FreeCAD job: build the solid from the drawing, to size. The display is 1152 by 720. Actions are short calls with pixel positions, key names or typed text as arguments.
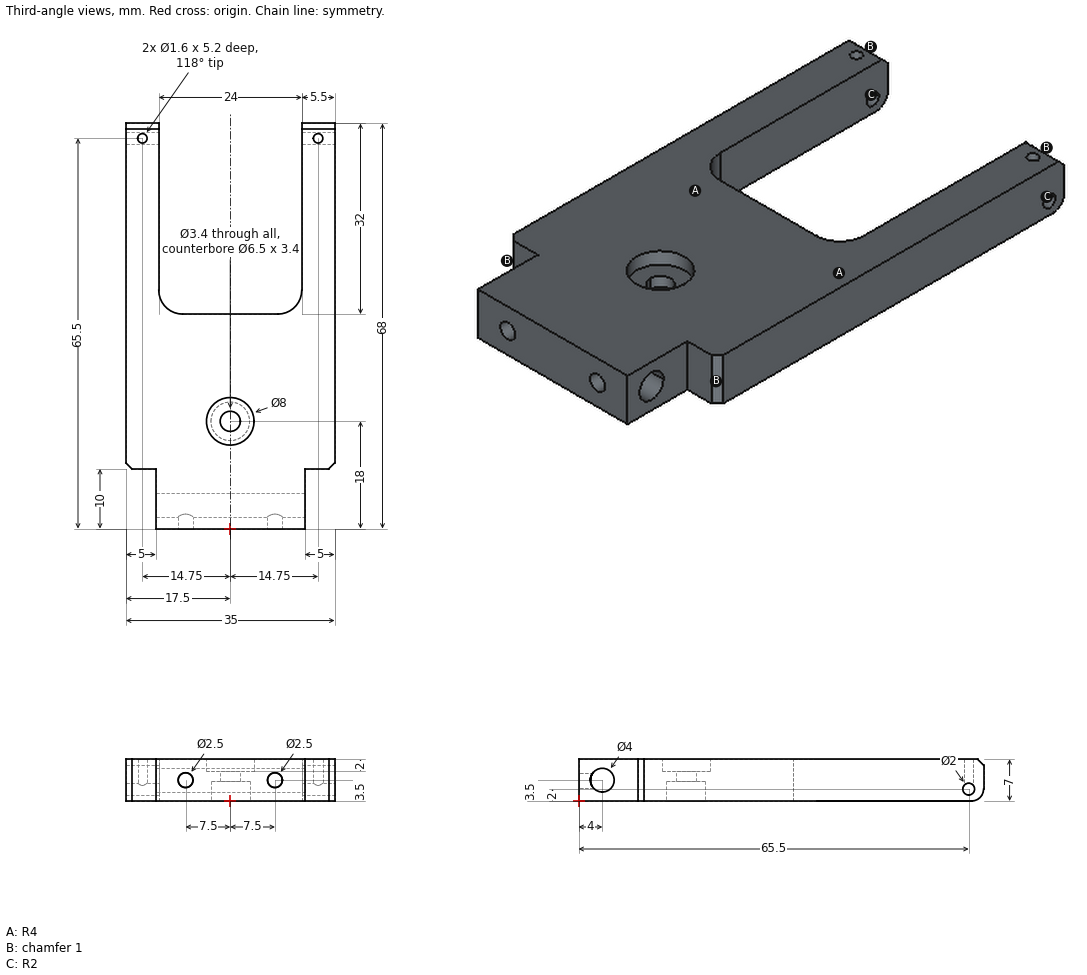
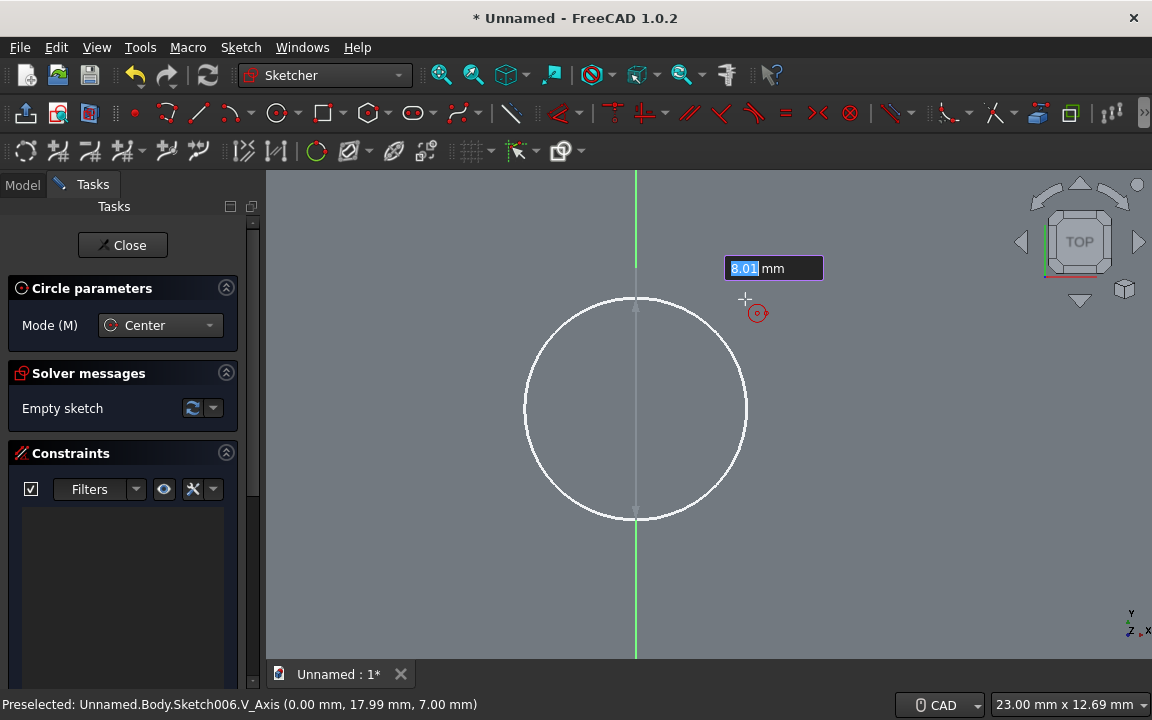
text(8)
key(Return)
key(Escape)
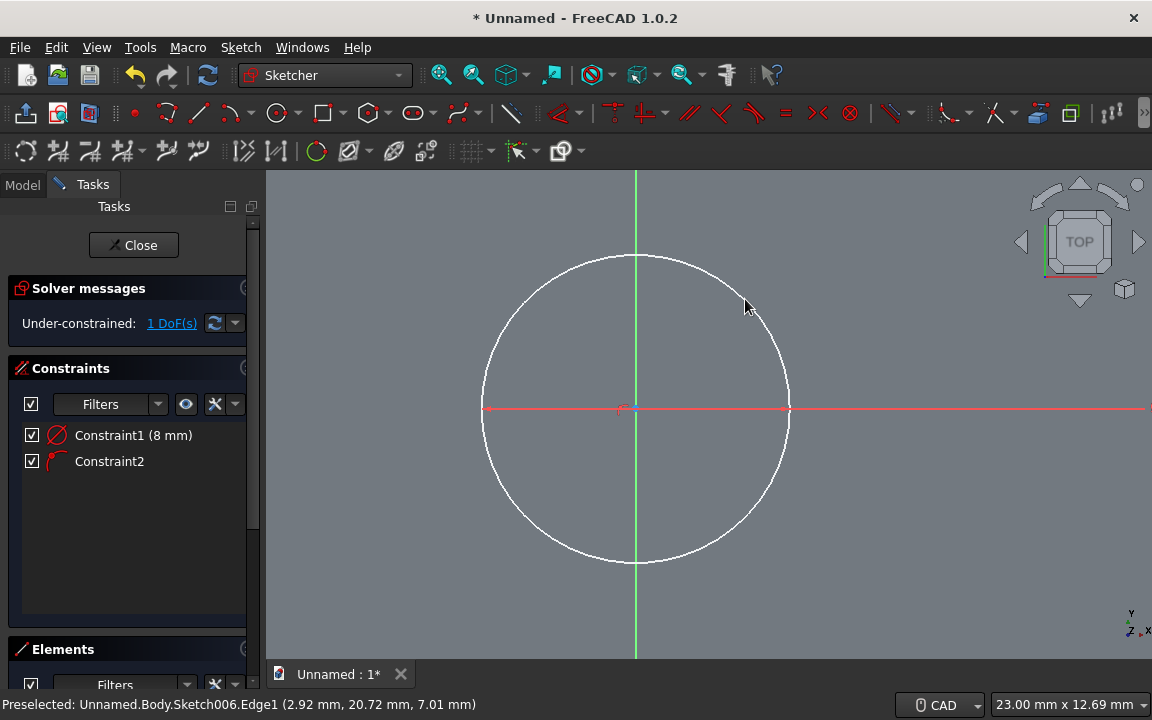
key(d)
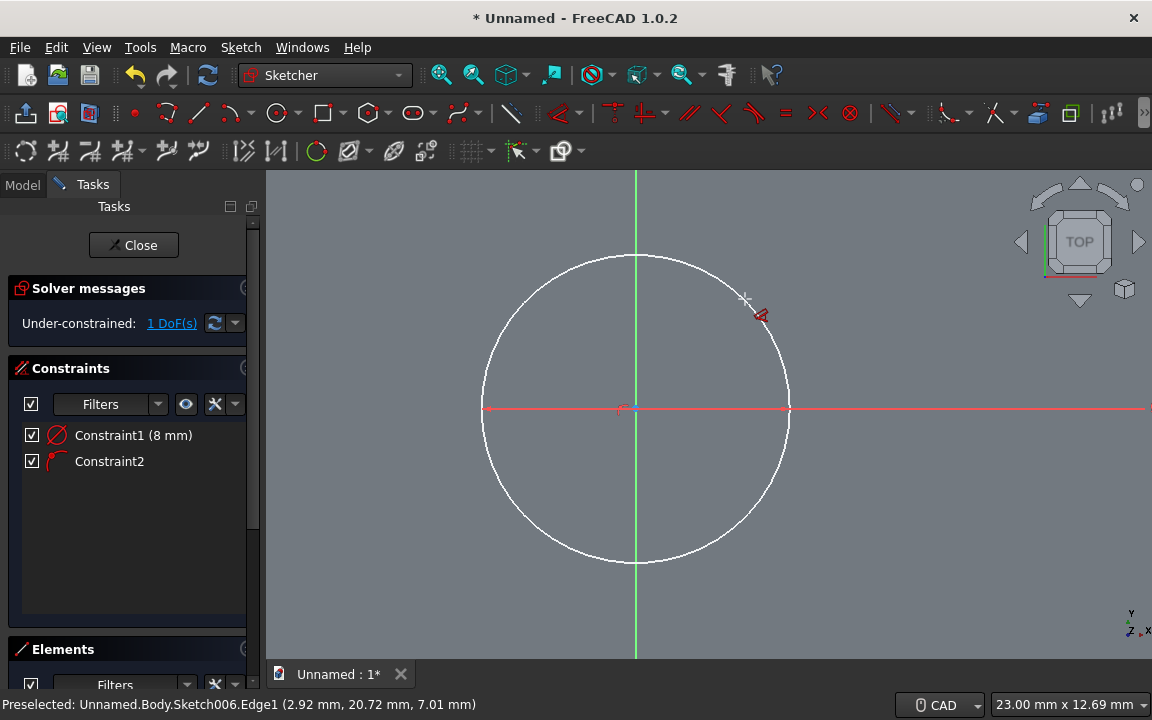
click(636, 409)
click(670, 520)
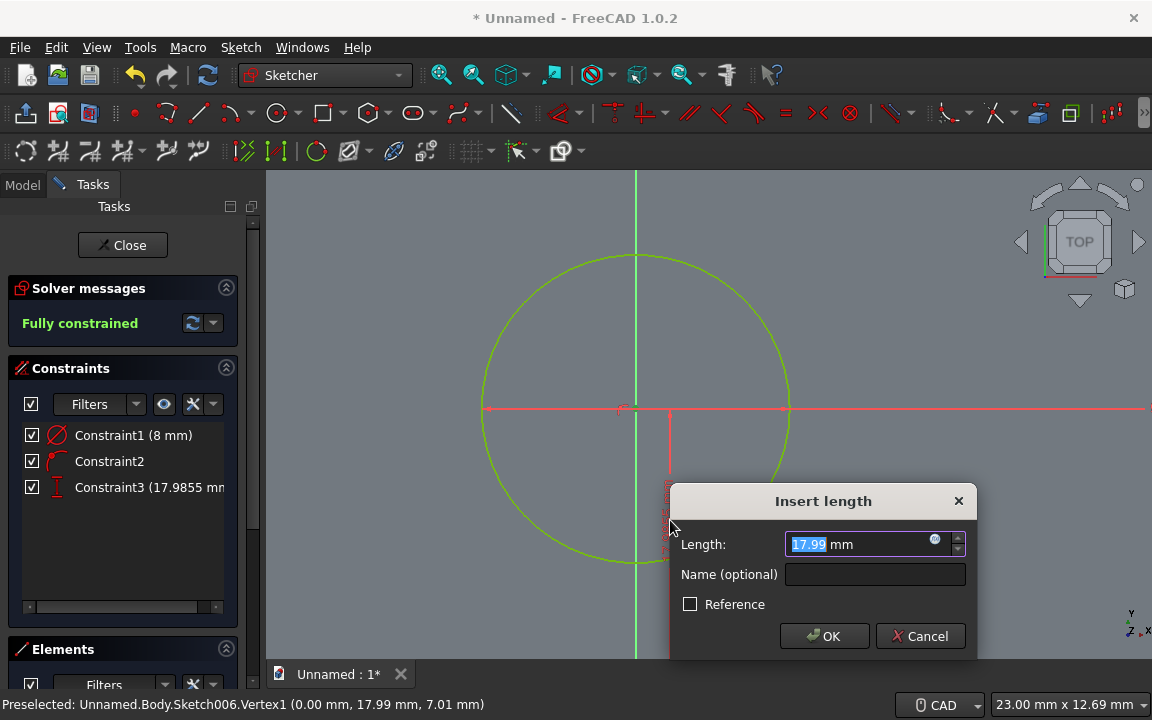
text(18)
key(Return)
key(Escape)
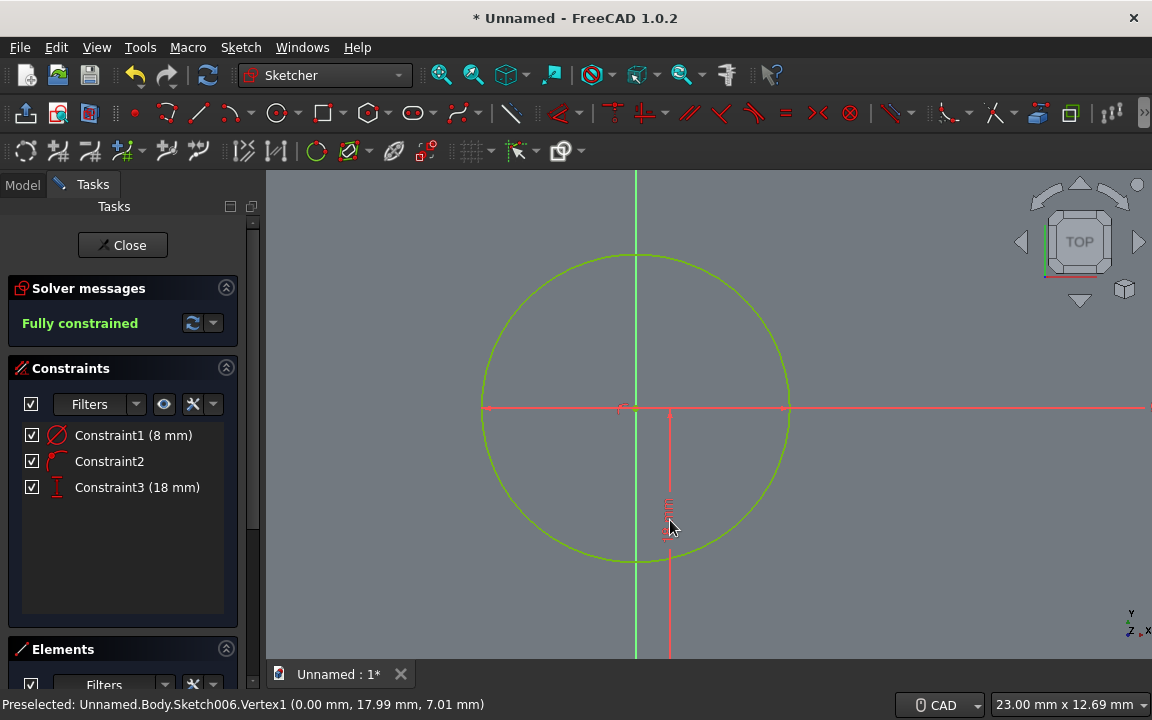
click(123, 245)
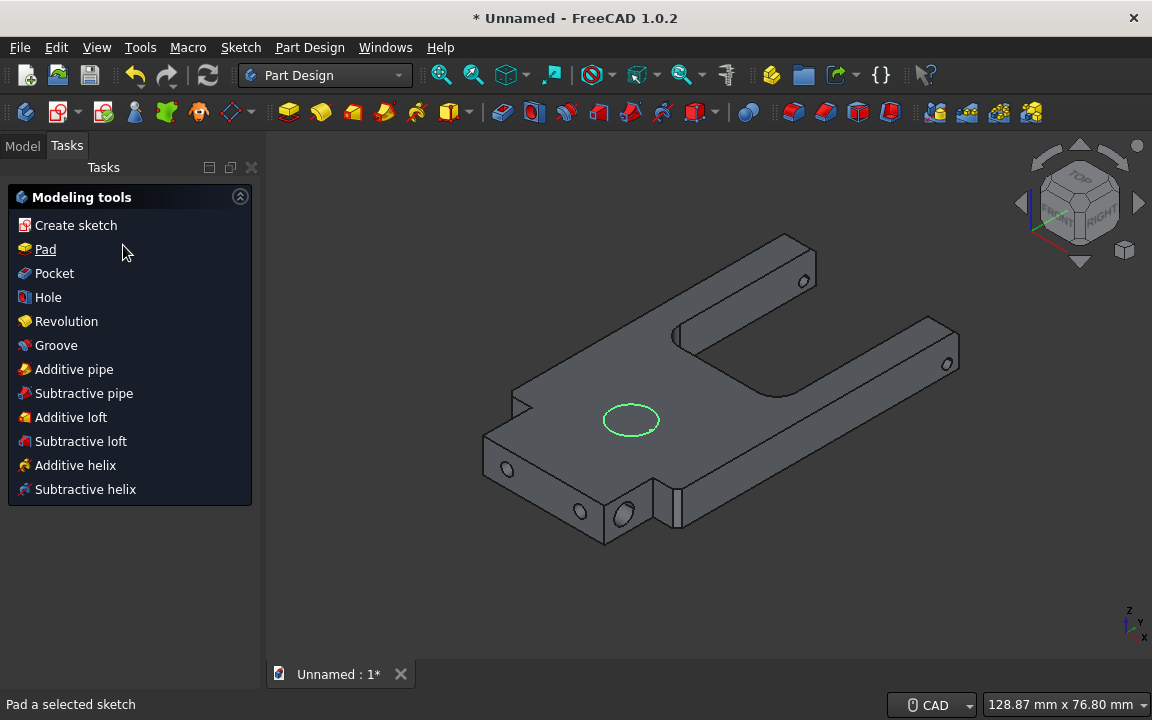
click(504, 112)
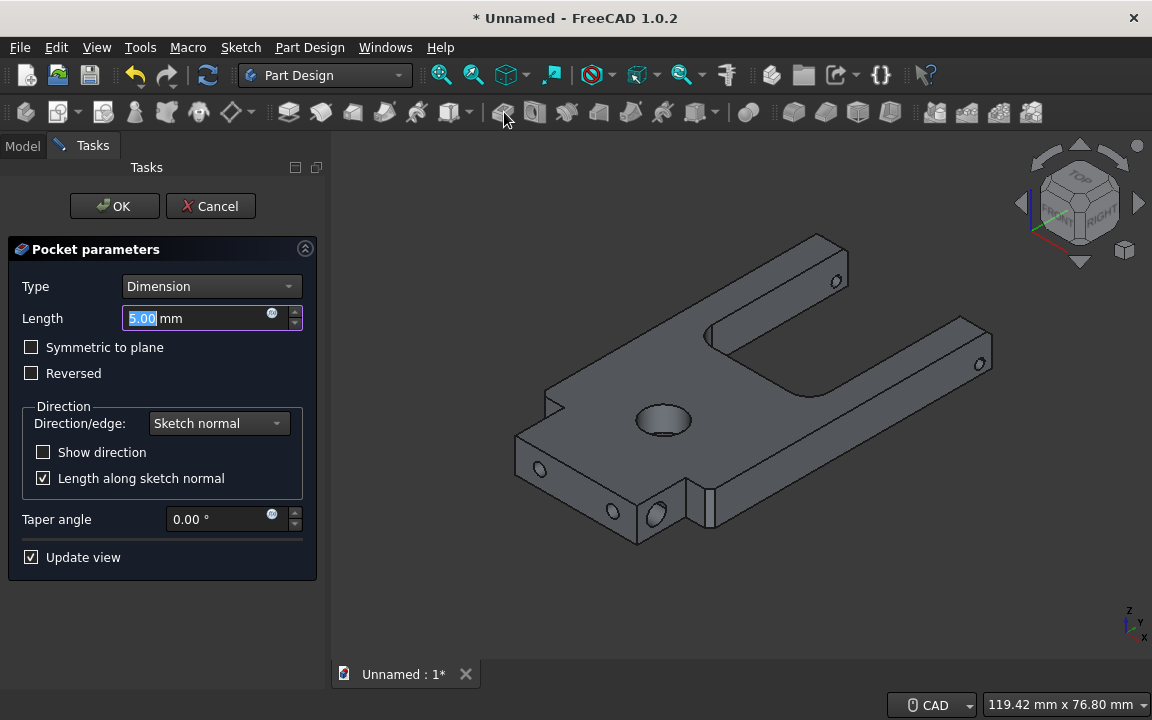
text(2)
key(Tab)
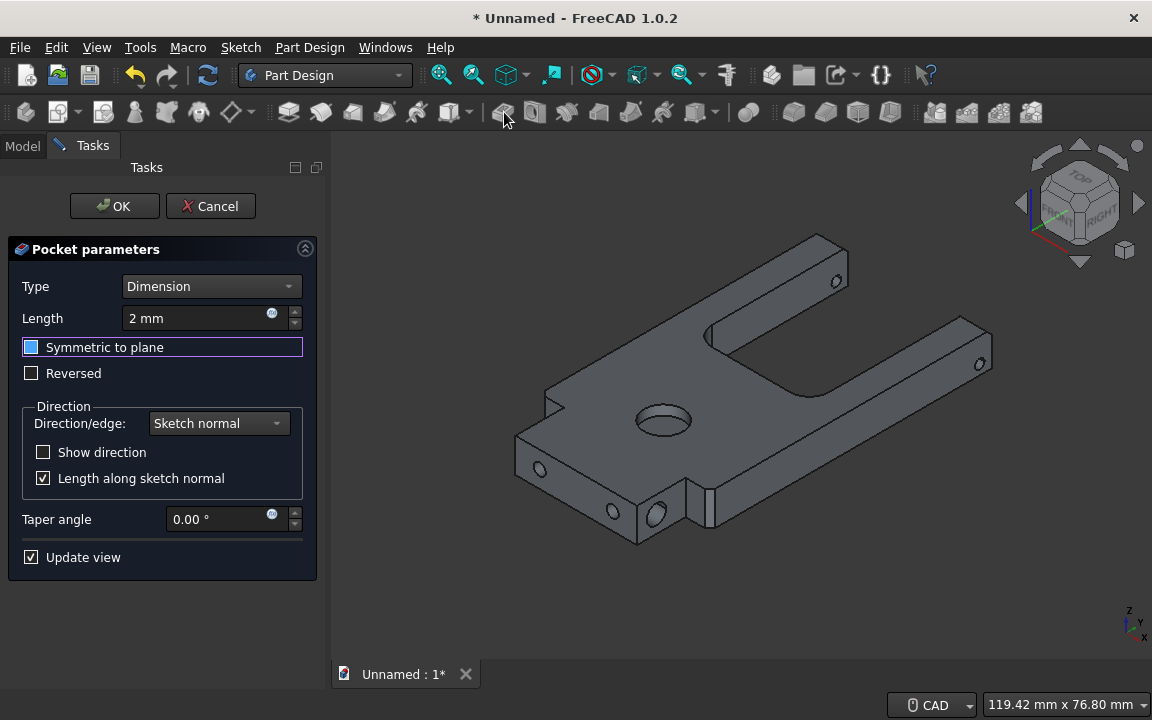
click(115, 206)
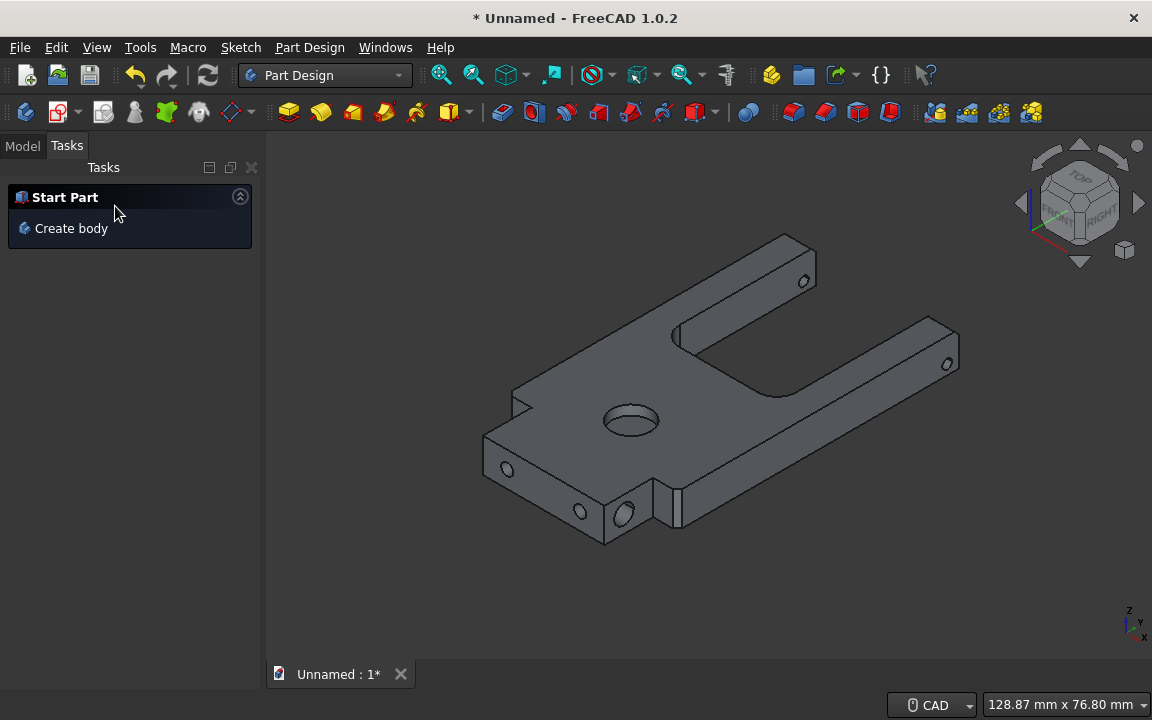
key(2)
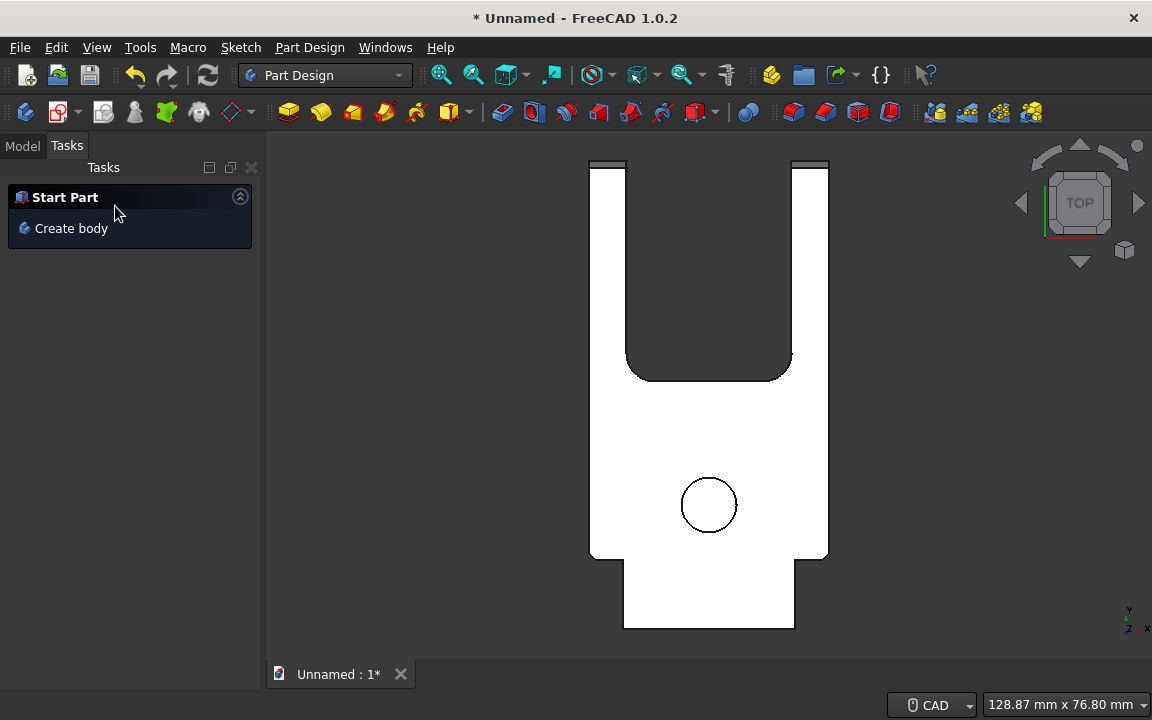
key(0)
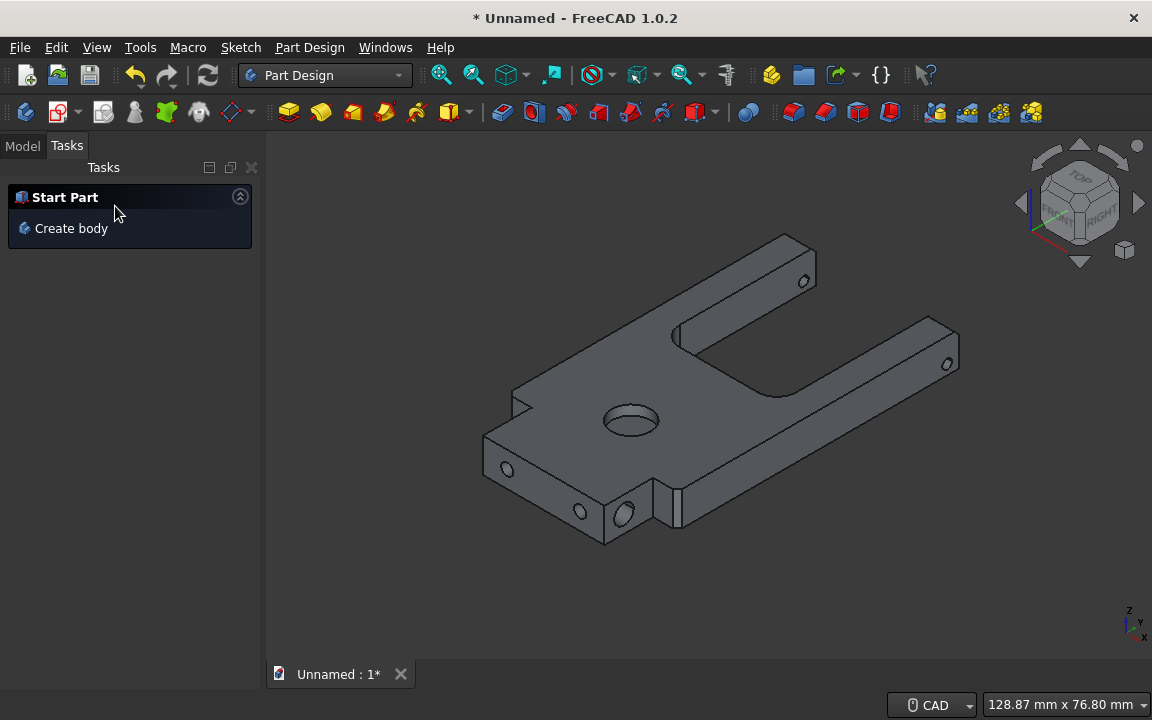
key(1)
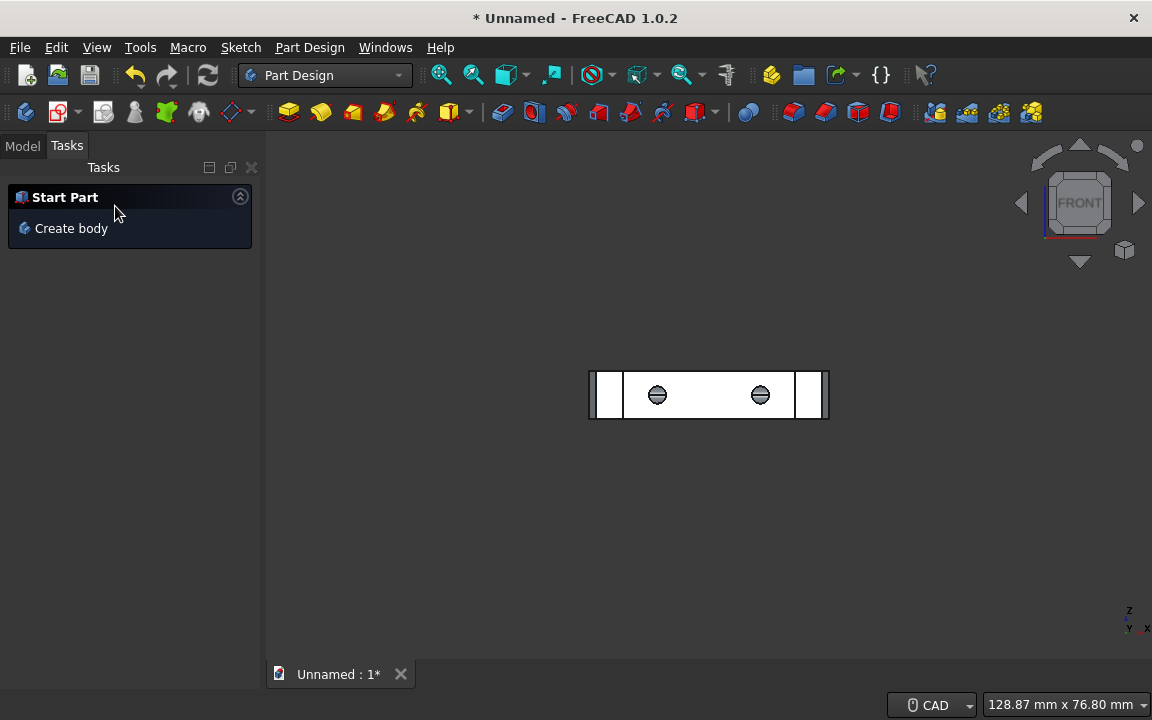
click(442, 76)